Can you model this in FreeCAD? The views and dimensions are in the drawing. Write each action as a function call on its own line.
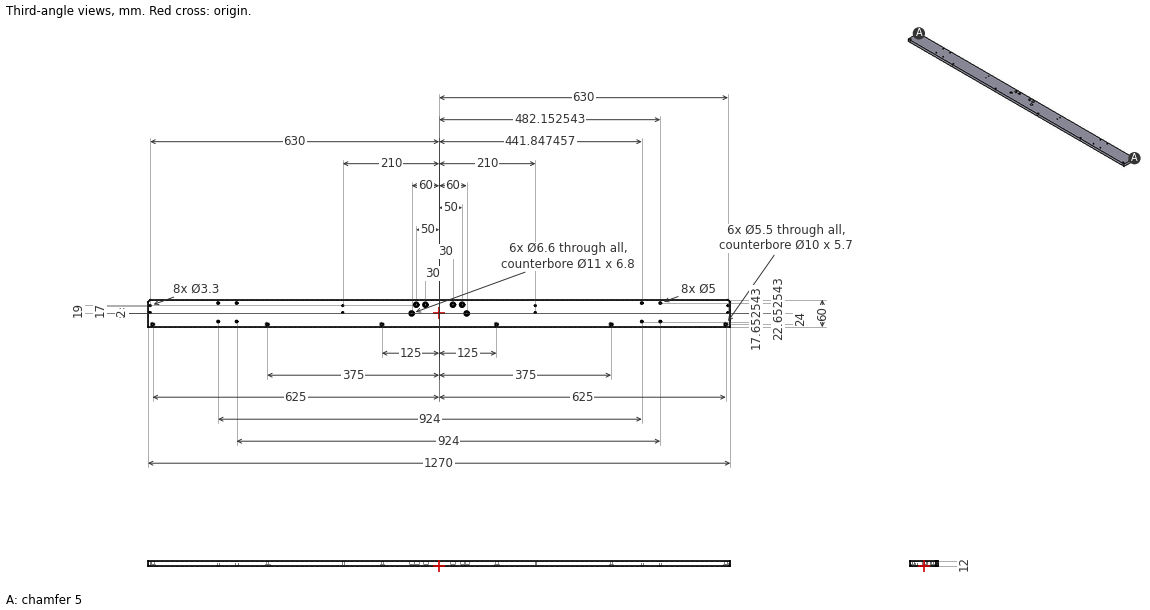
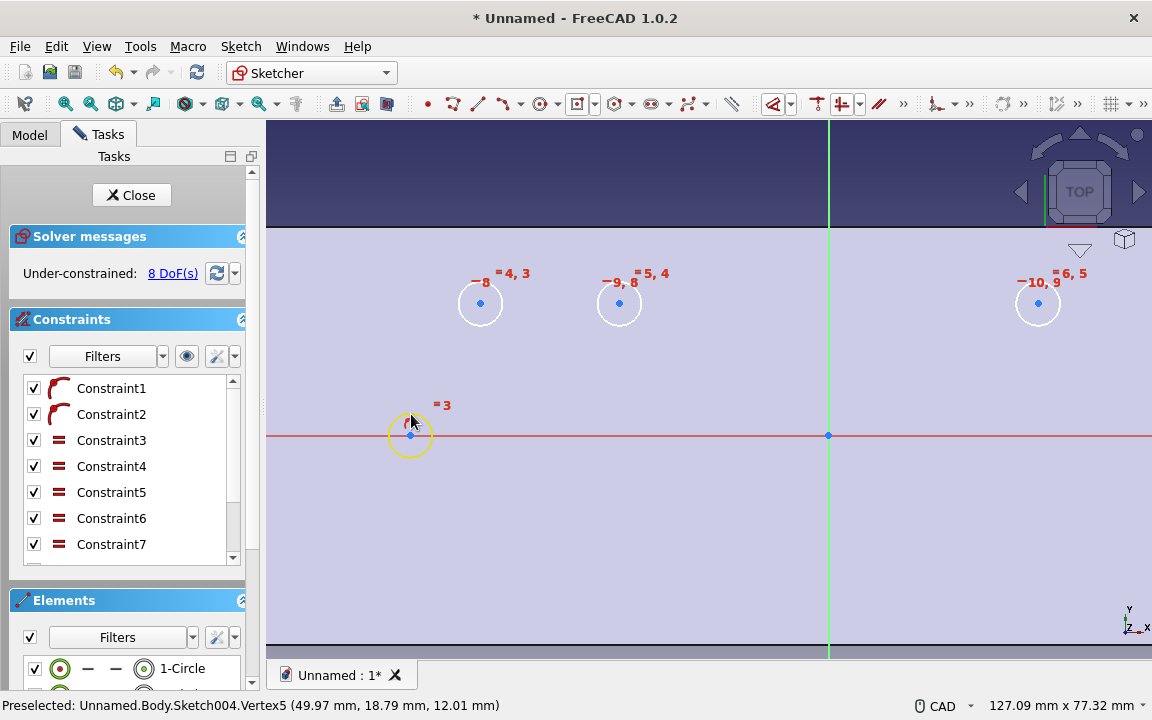
click(411, 414)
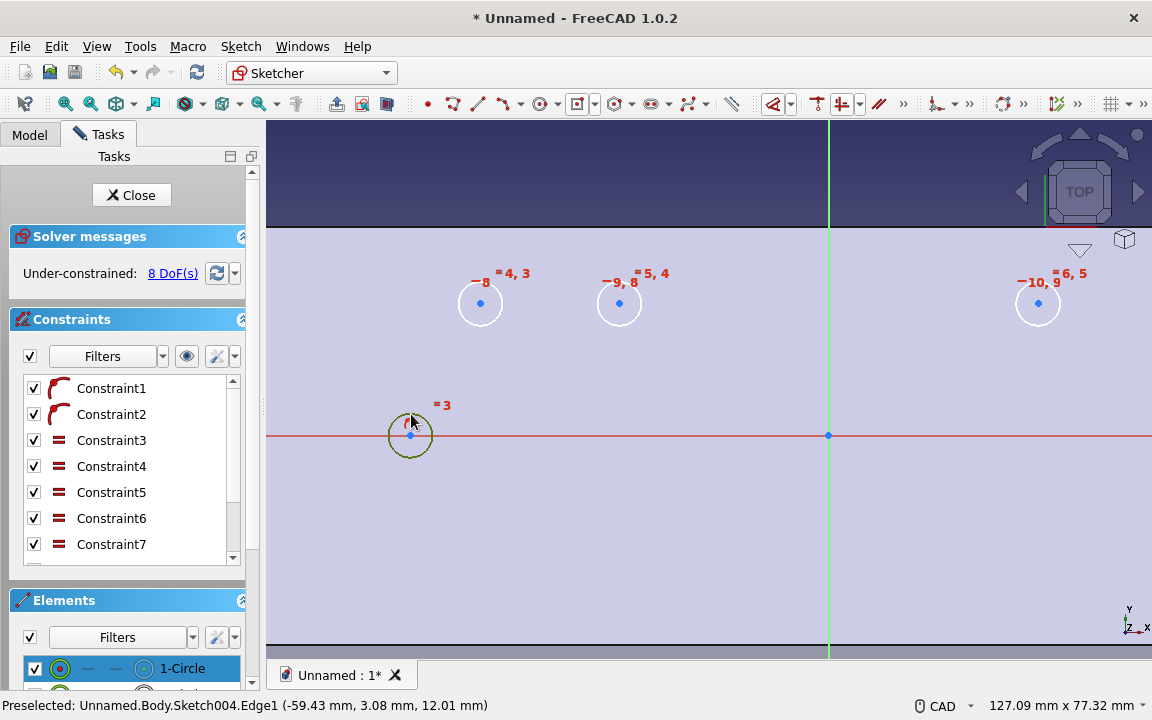
key(k)
key(o)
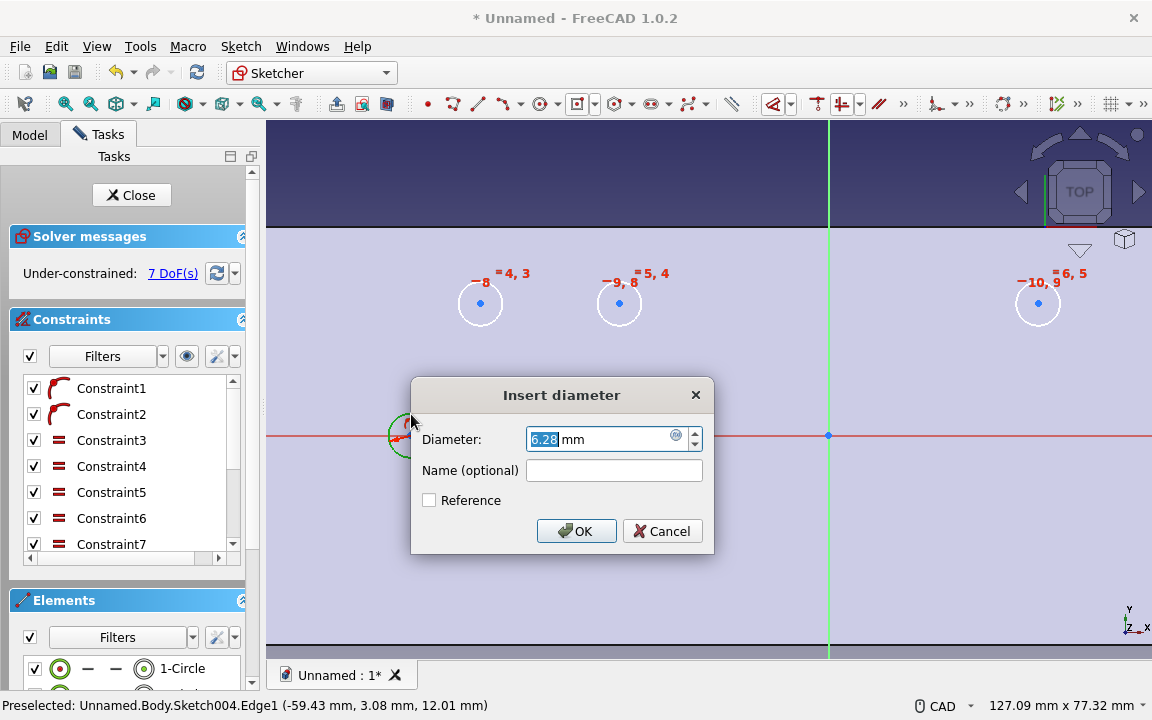
text(6.6)
key(Return)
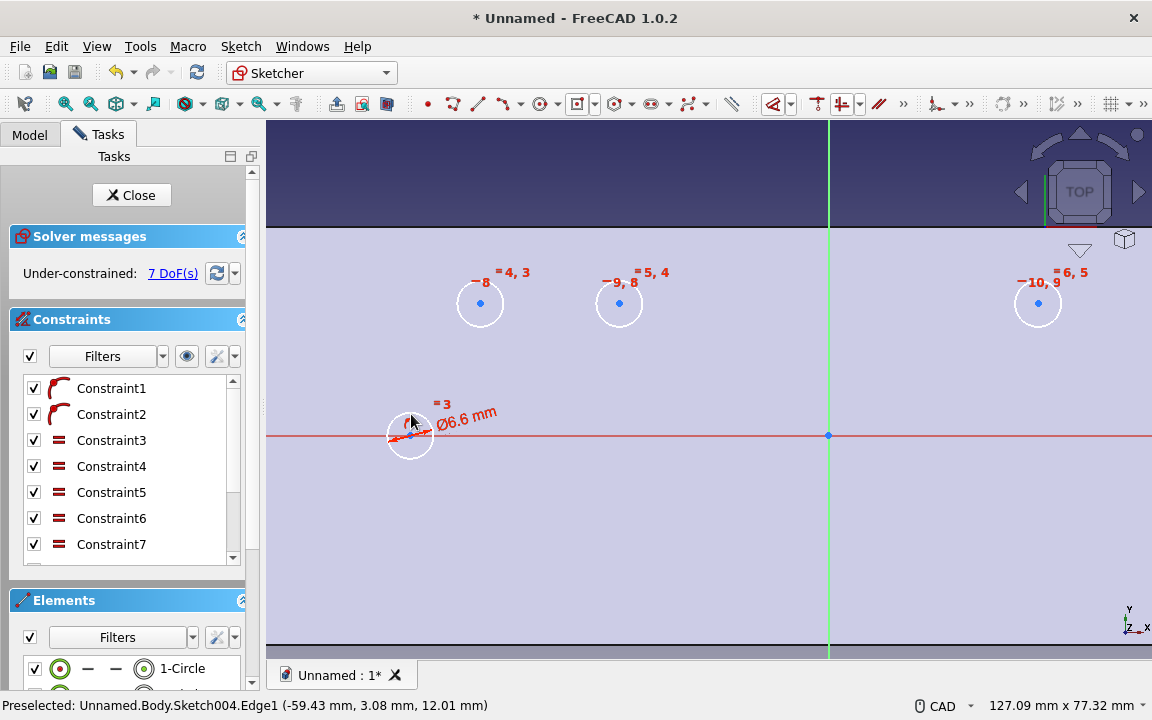
click(410, 436)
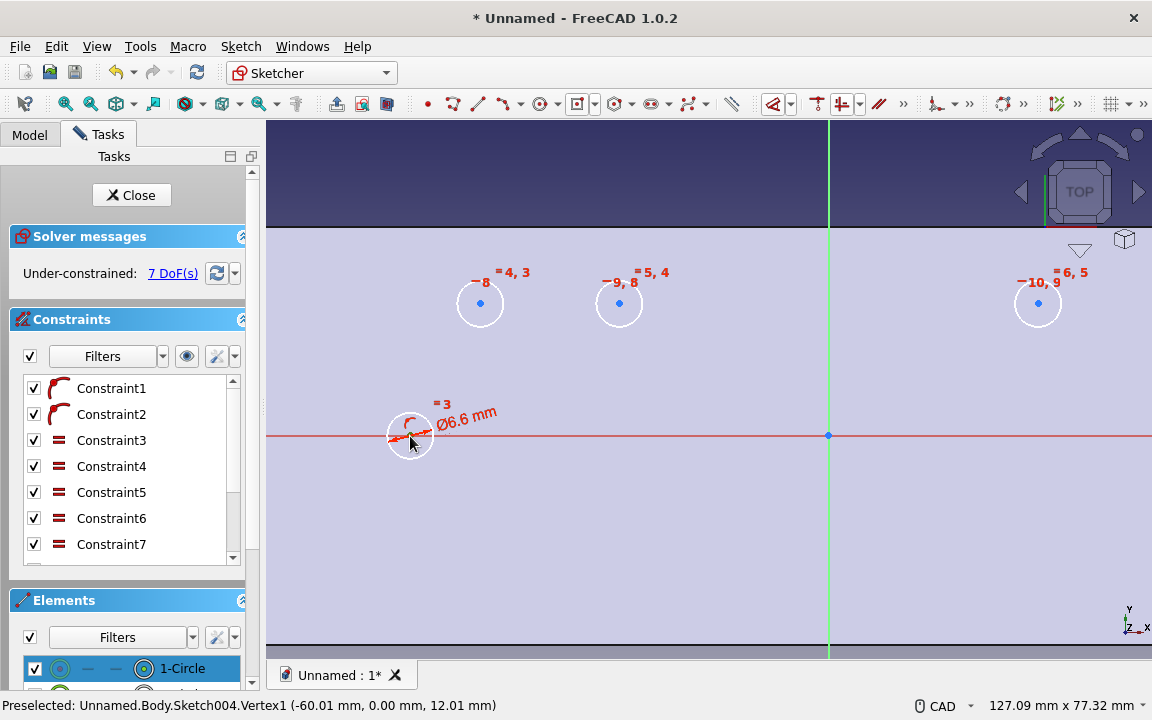
click(790, 104)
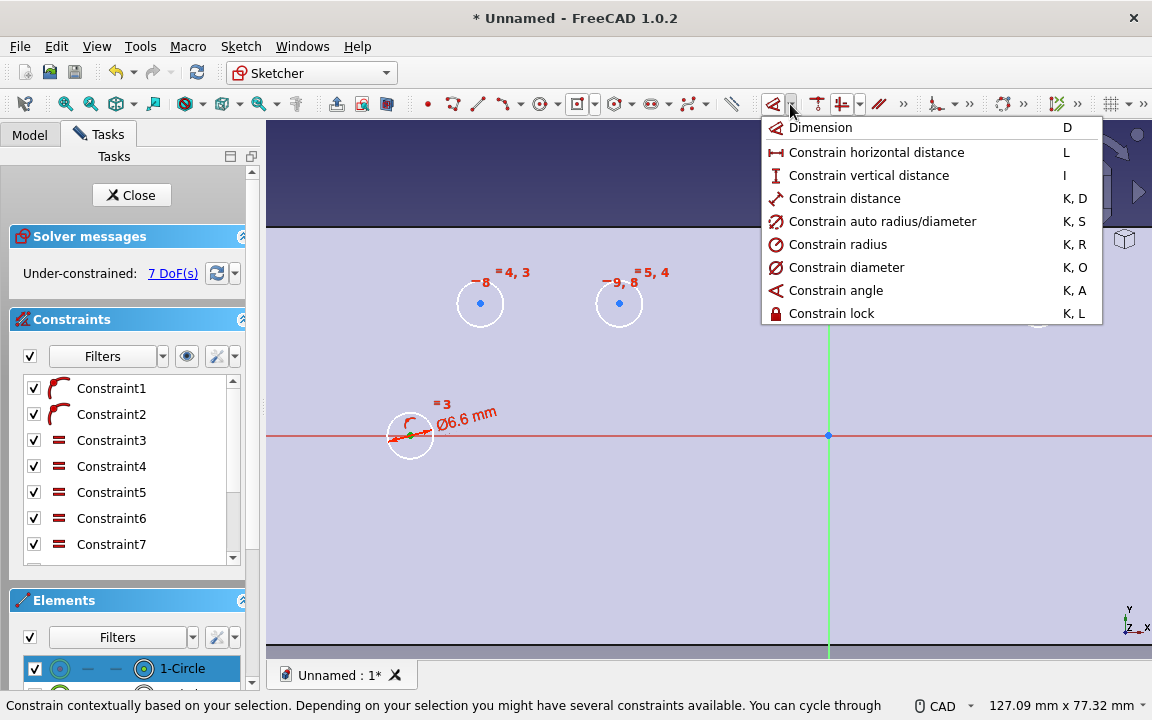
click(932, 152)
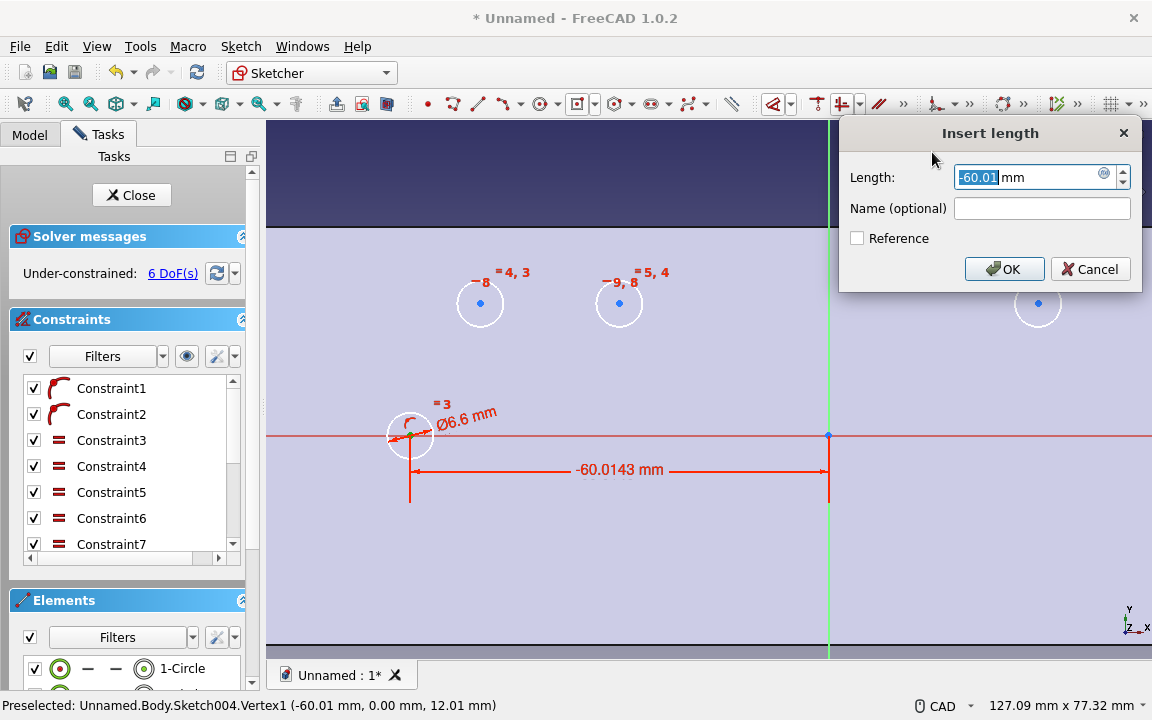
text(-60)
key(Return)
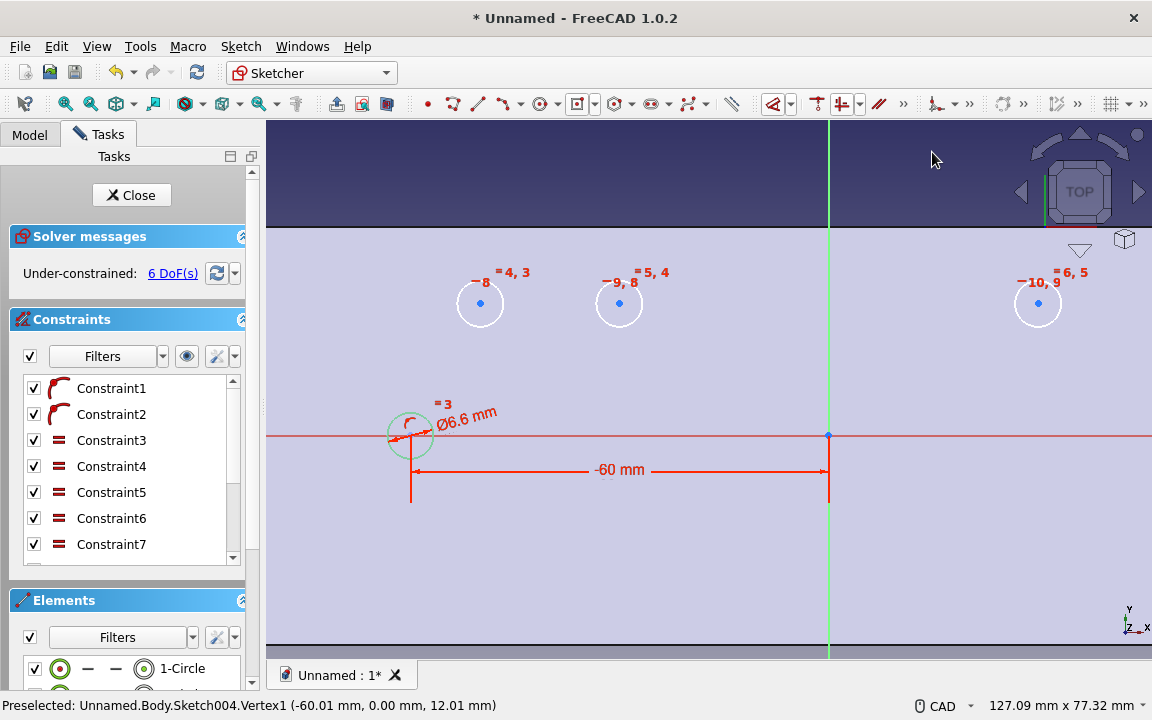
click(480, 304)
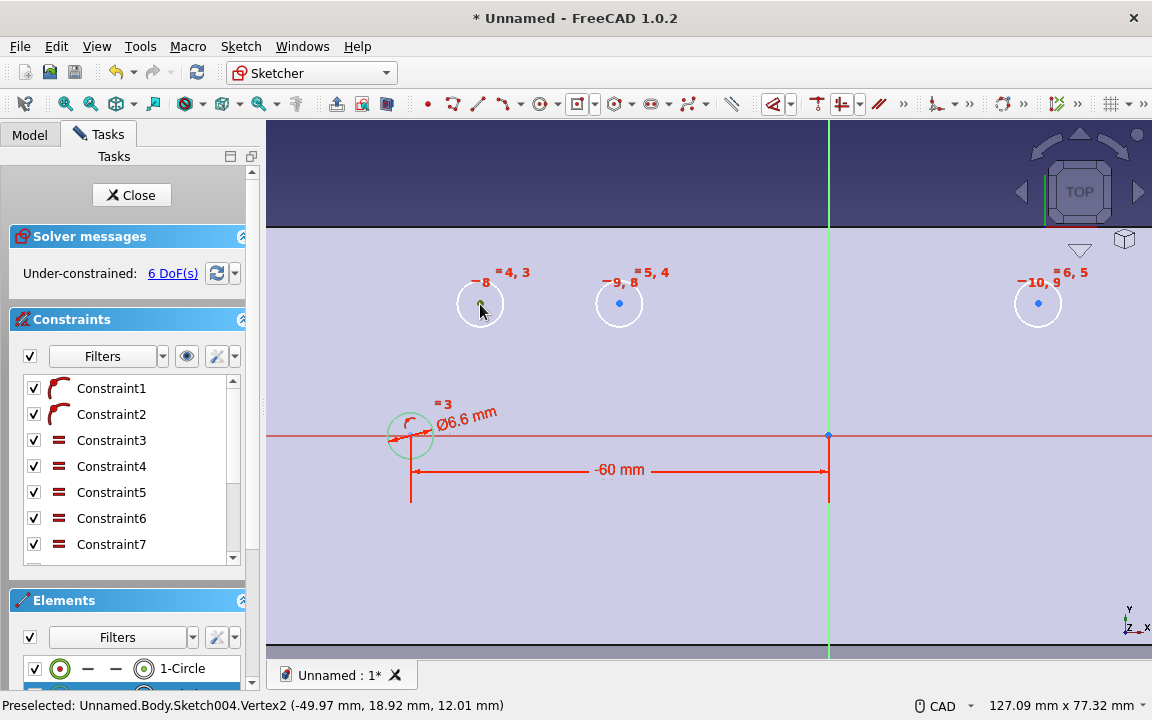
key(l)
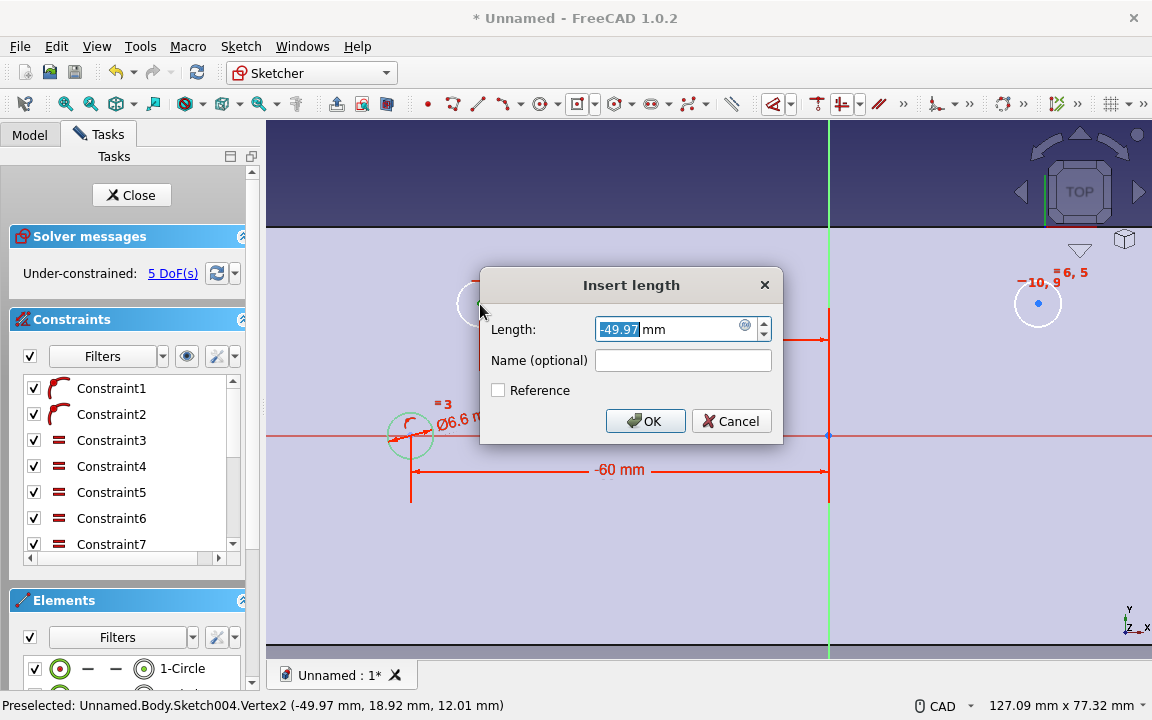
text(-50)
key(Return)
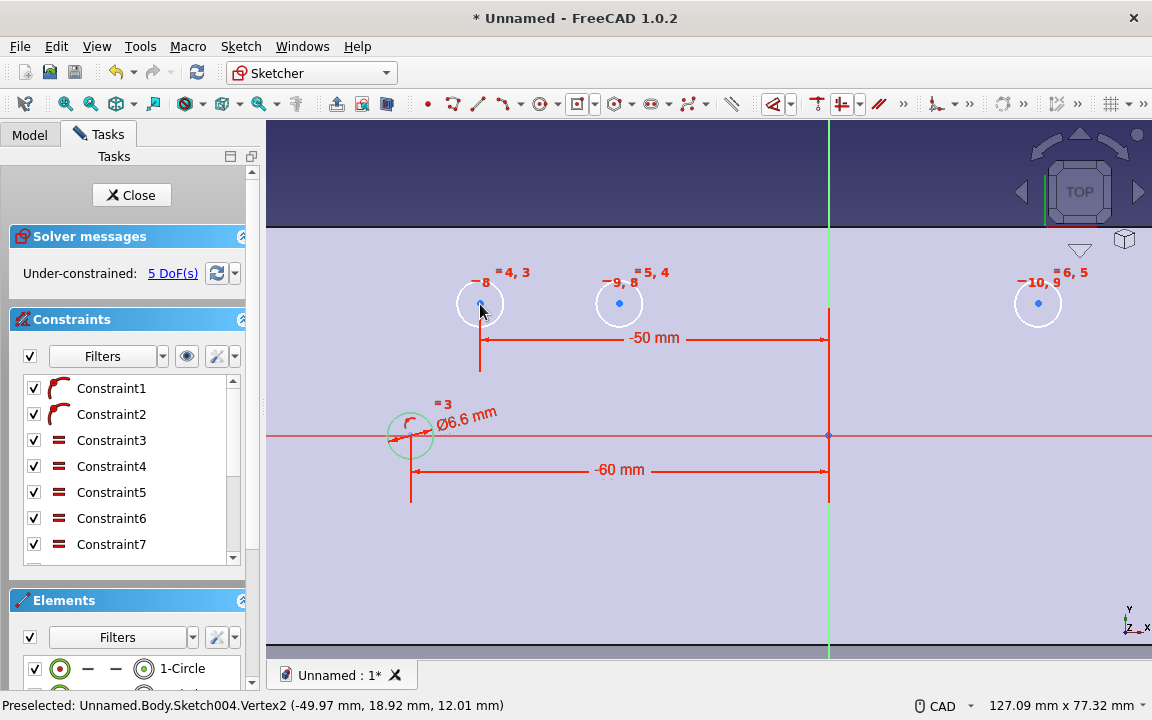
click(480, 304)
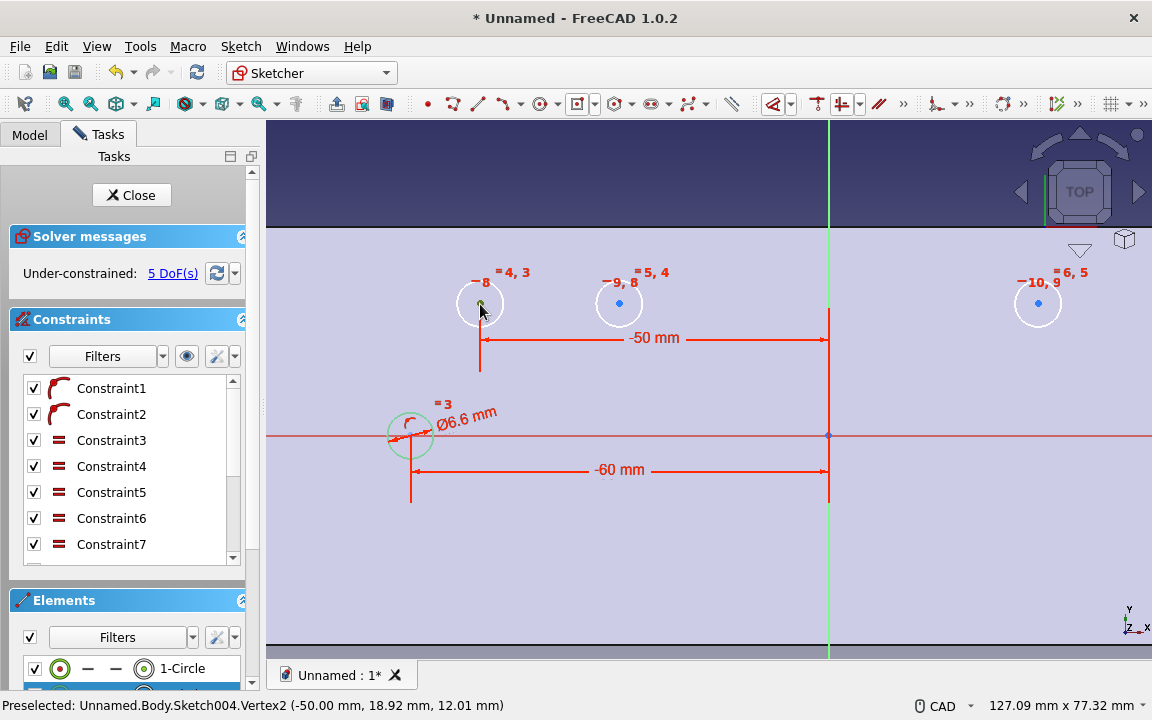
key(i)